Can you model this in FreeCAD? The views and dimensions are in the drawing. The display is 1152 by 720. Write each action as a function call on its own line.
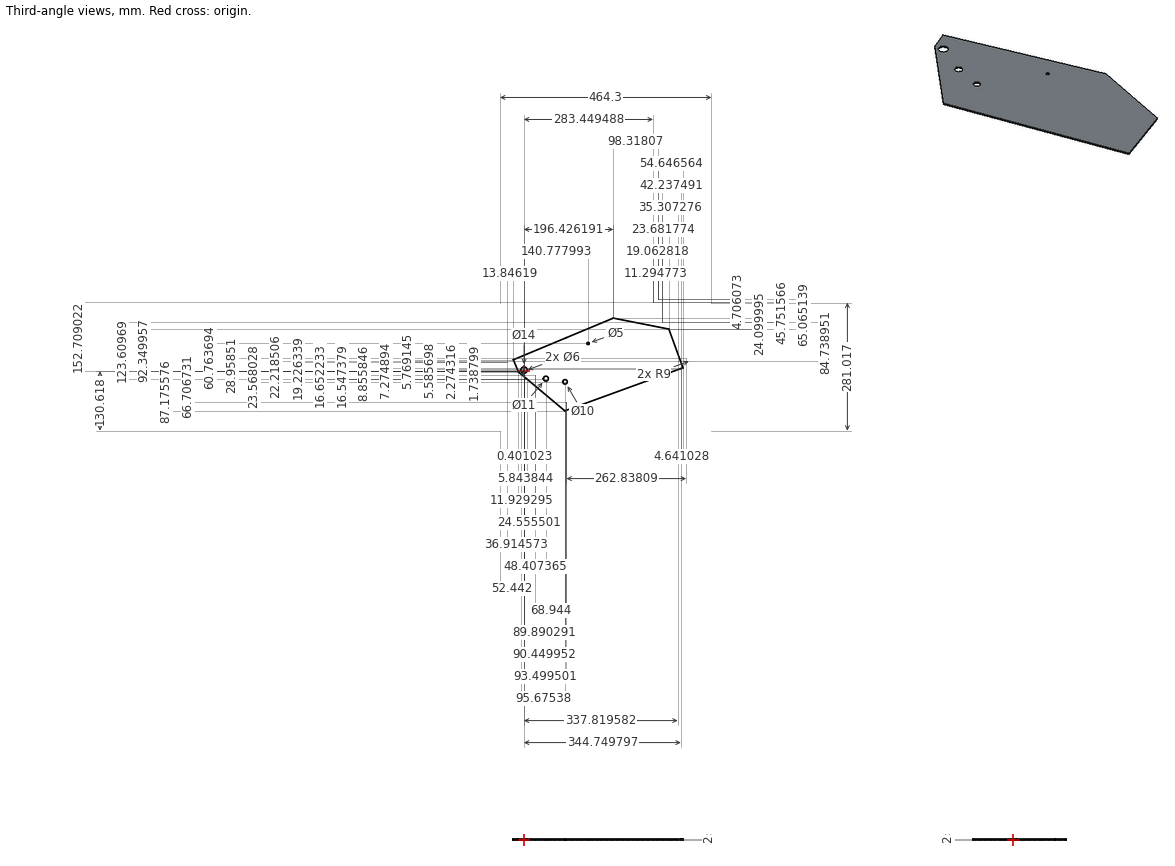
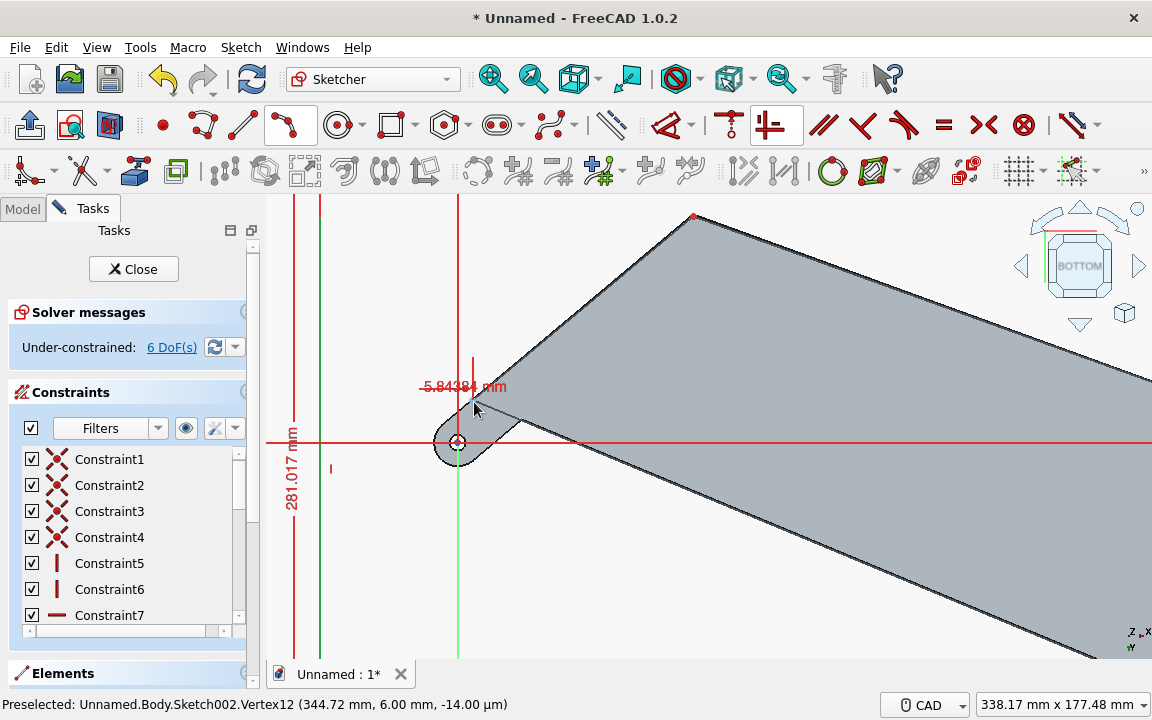
click(473, 400)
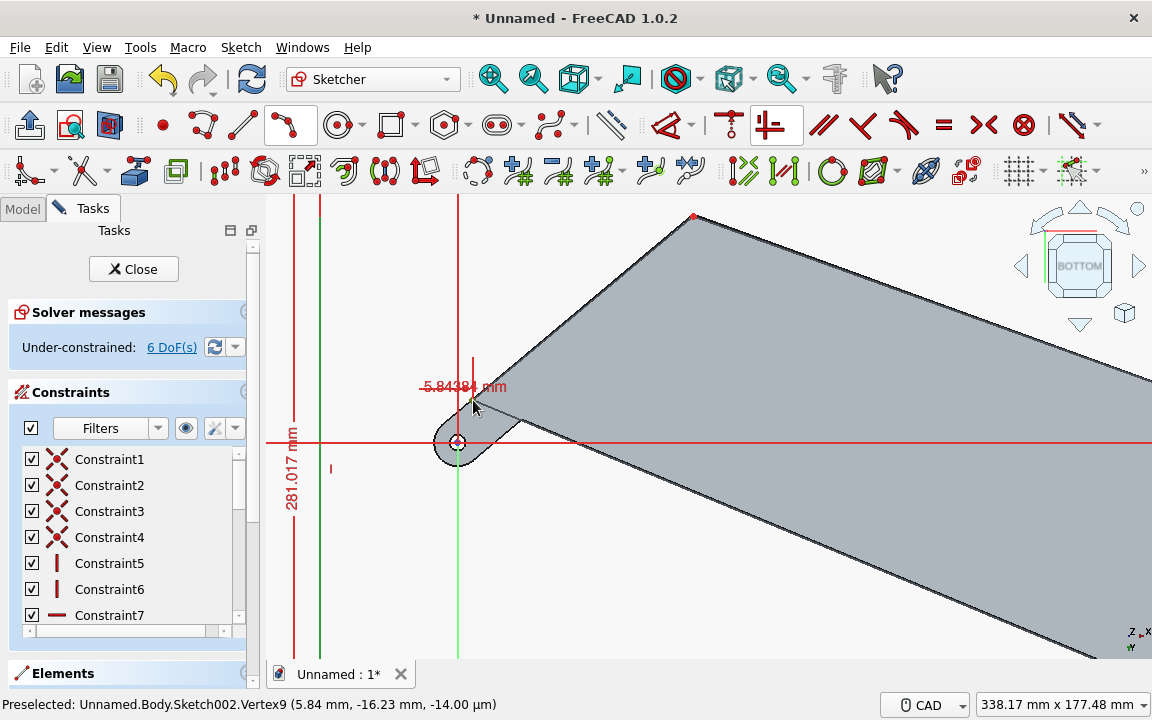
key(i)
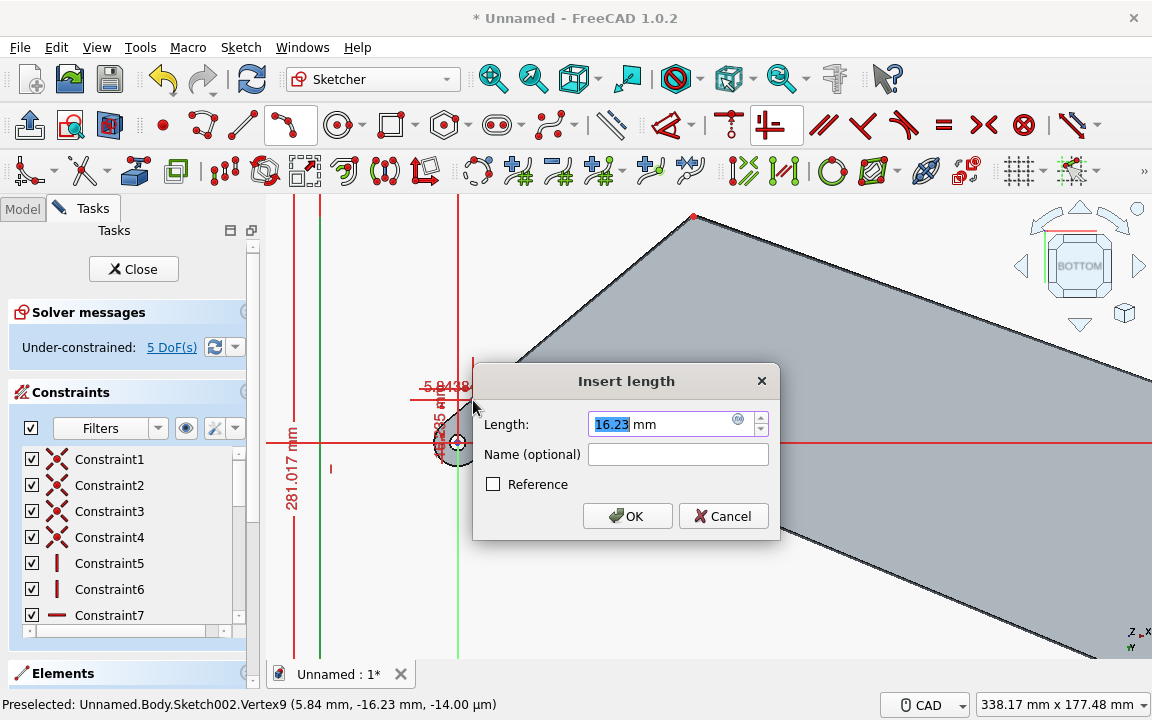
text(16.652233)
key(Return)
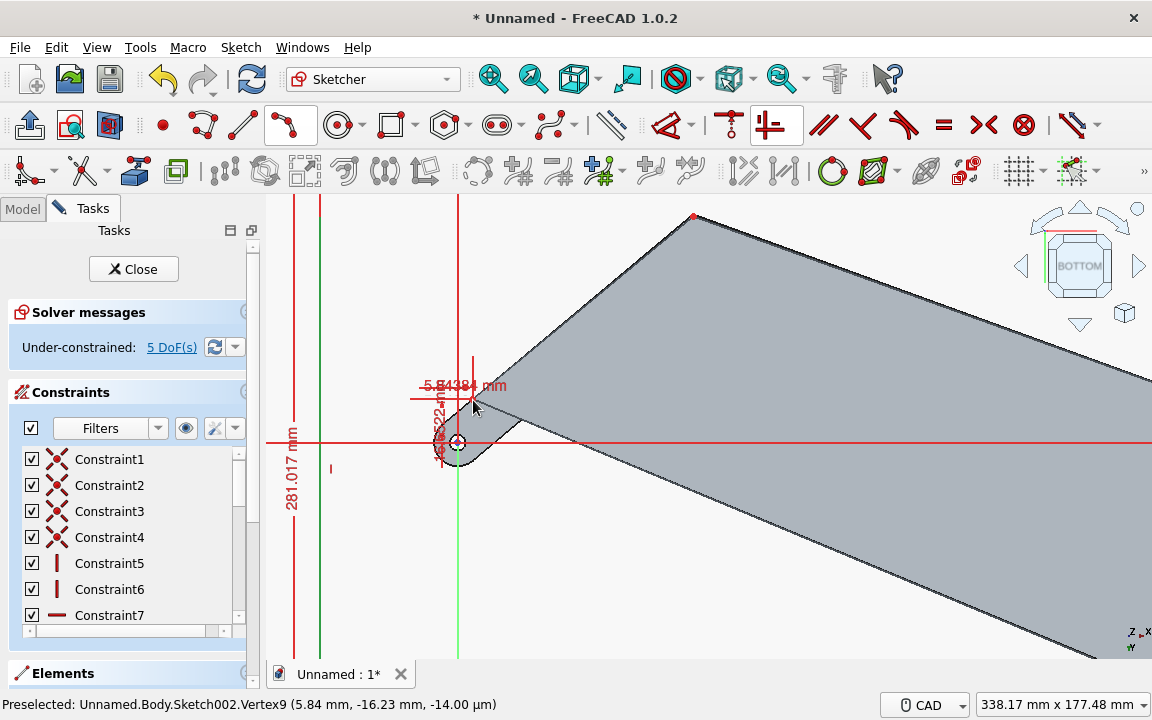
scroll(473, 402, down, 5)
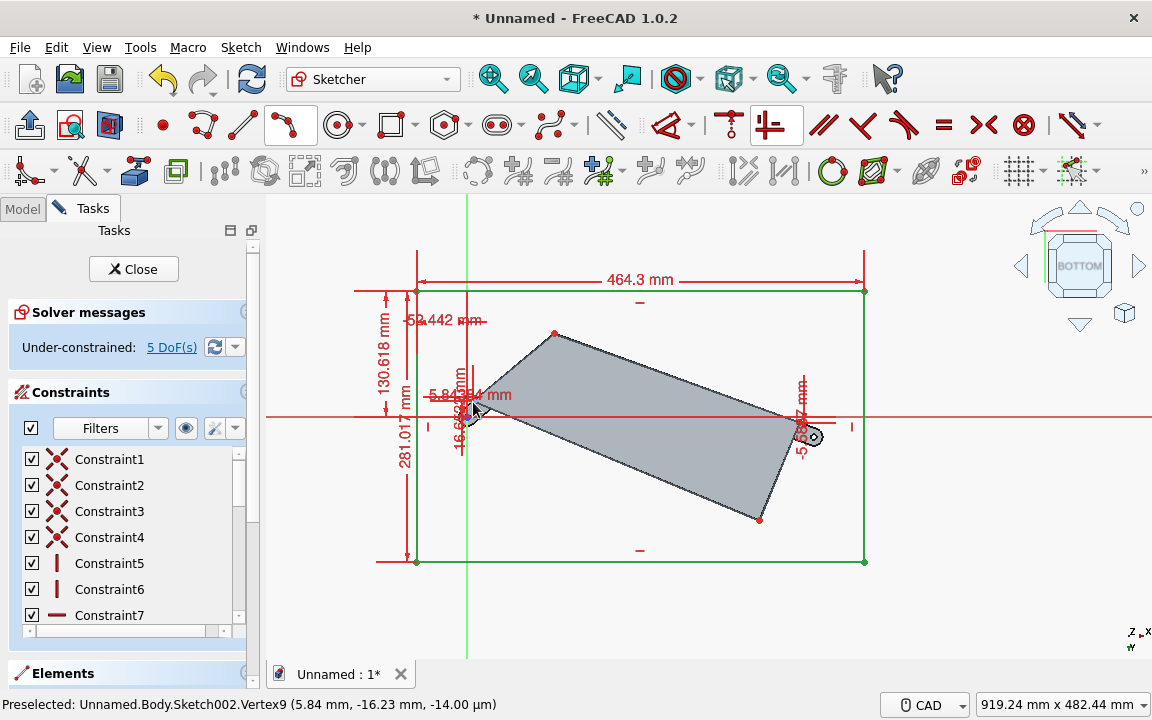
click(554, 334)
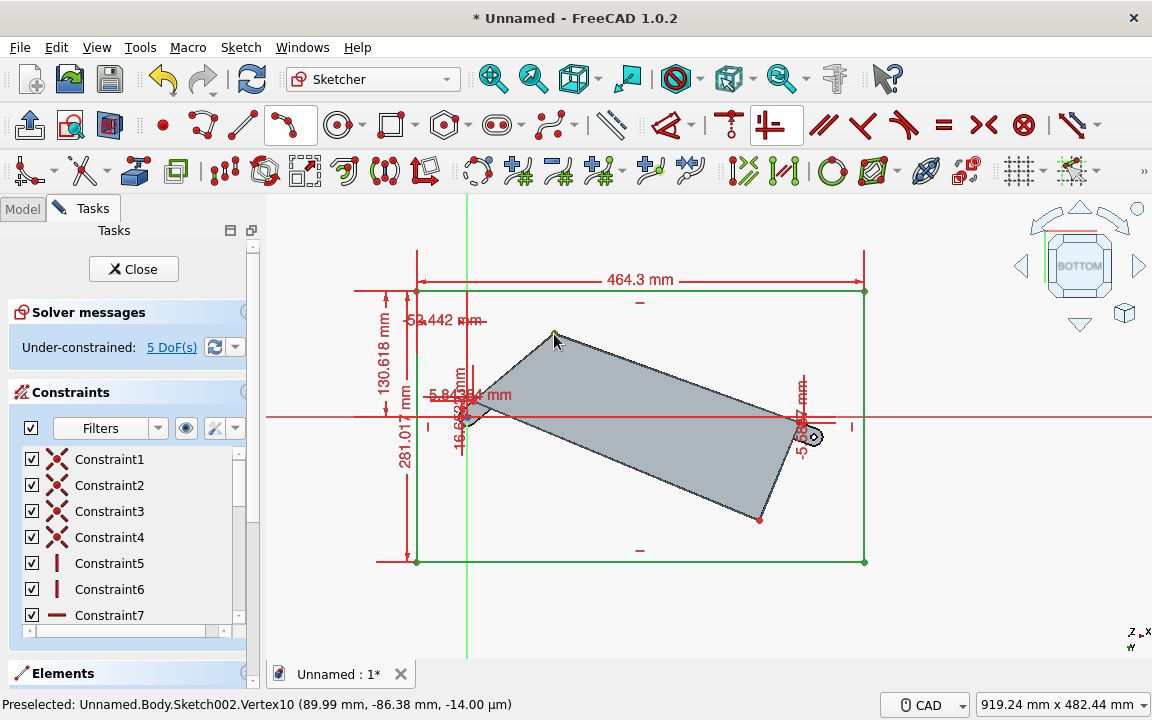
key(l)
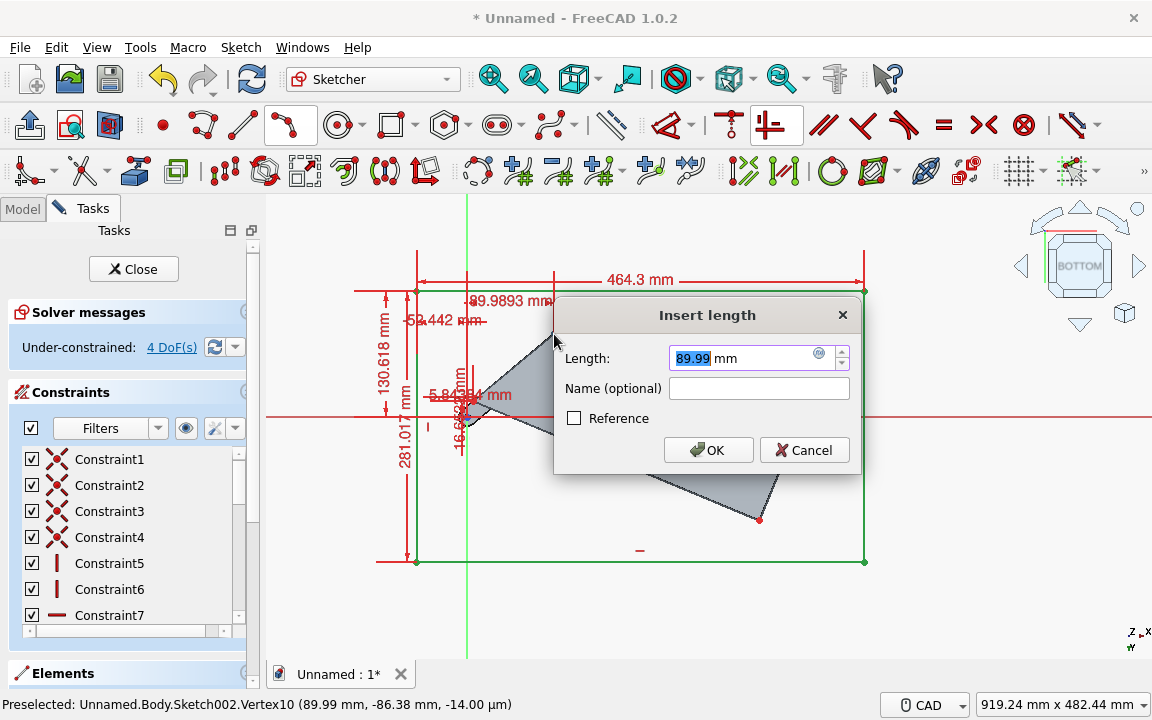
text(89.890291)
key(Return)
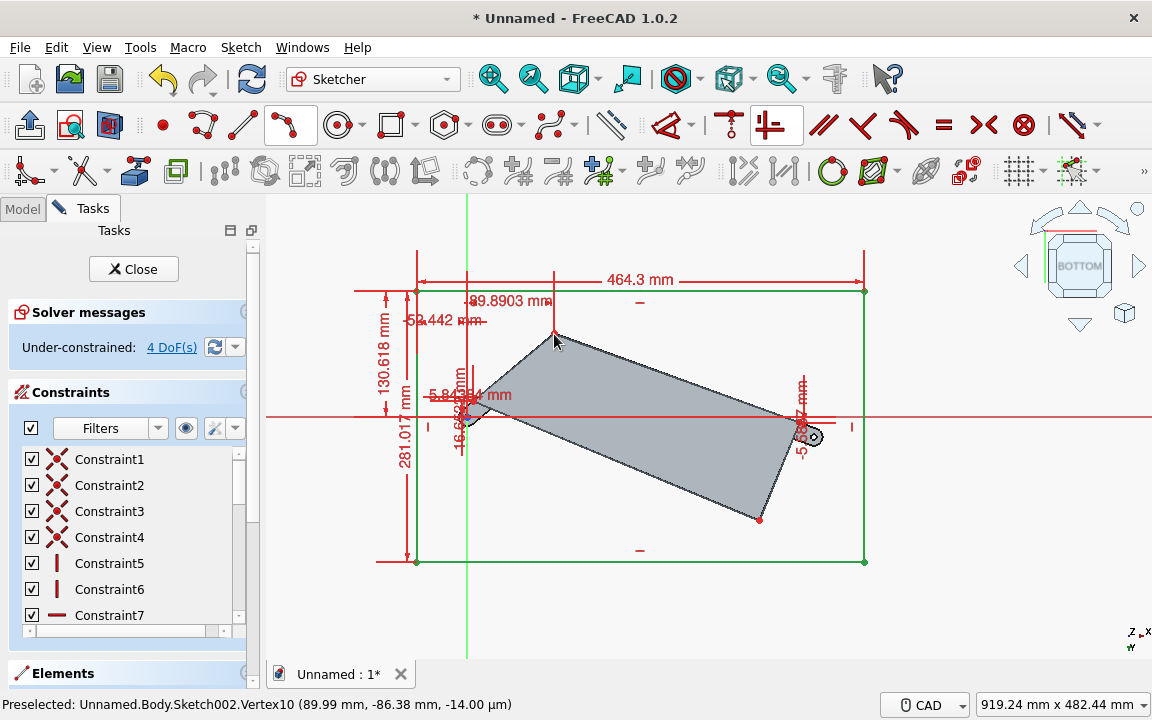
click(554, 334)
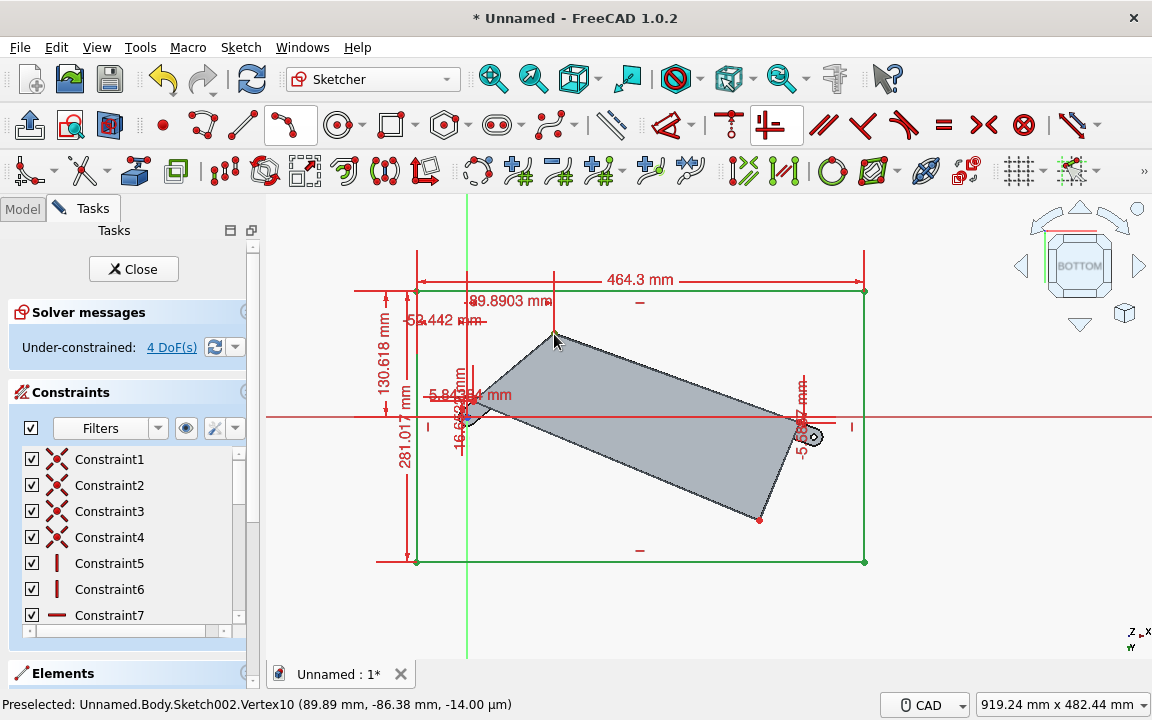
key(i)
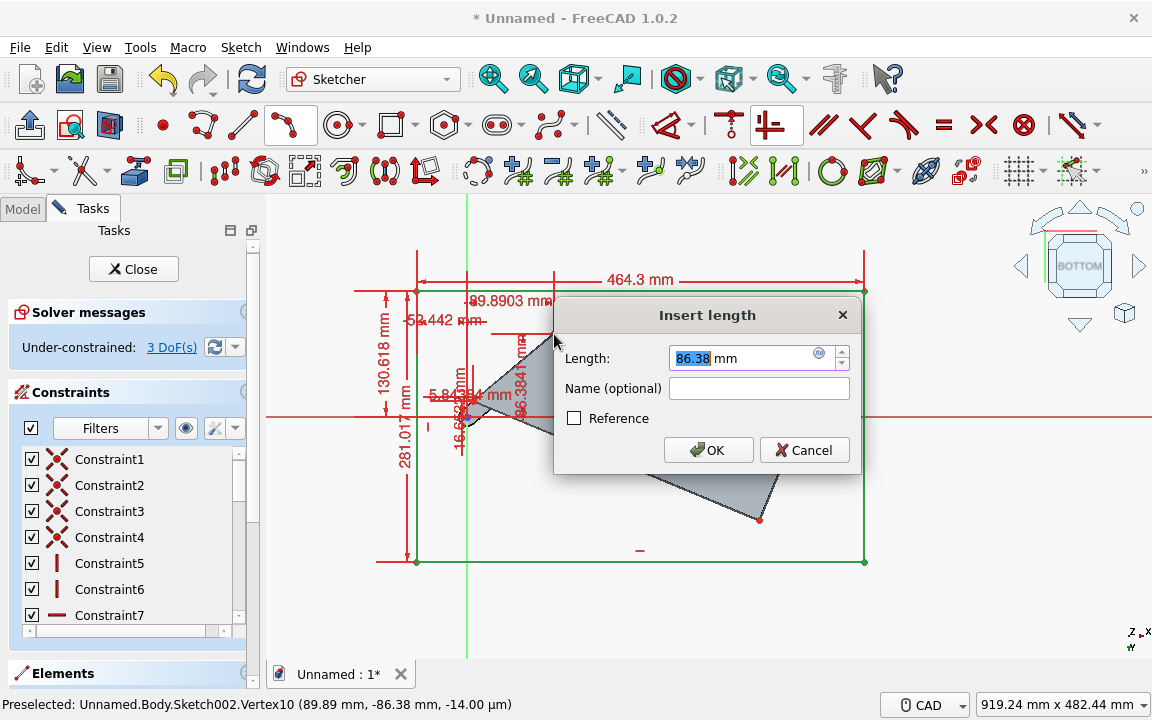
text(87.175576)
key(Return)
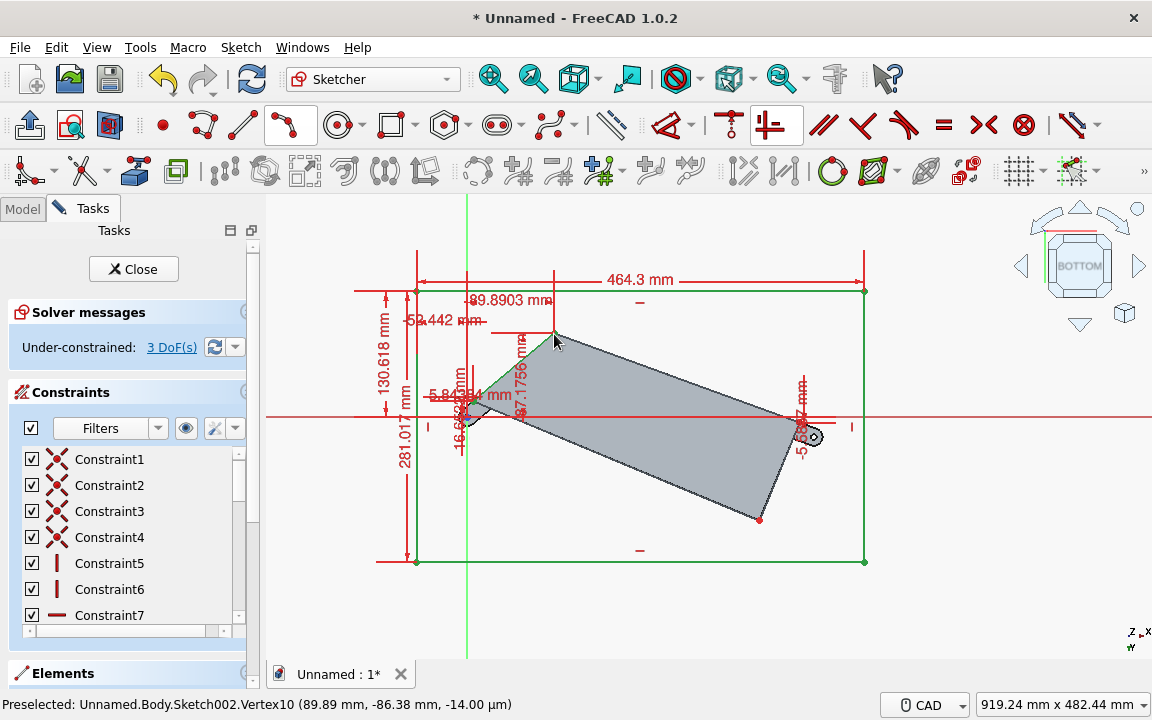
click(788, 452)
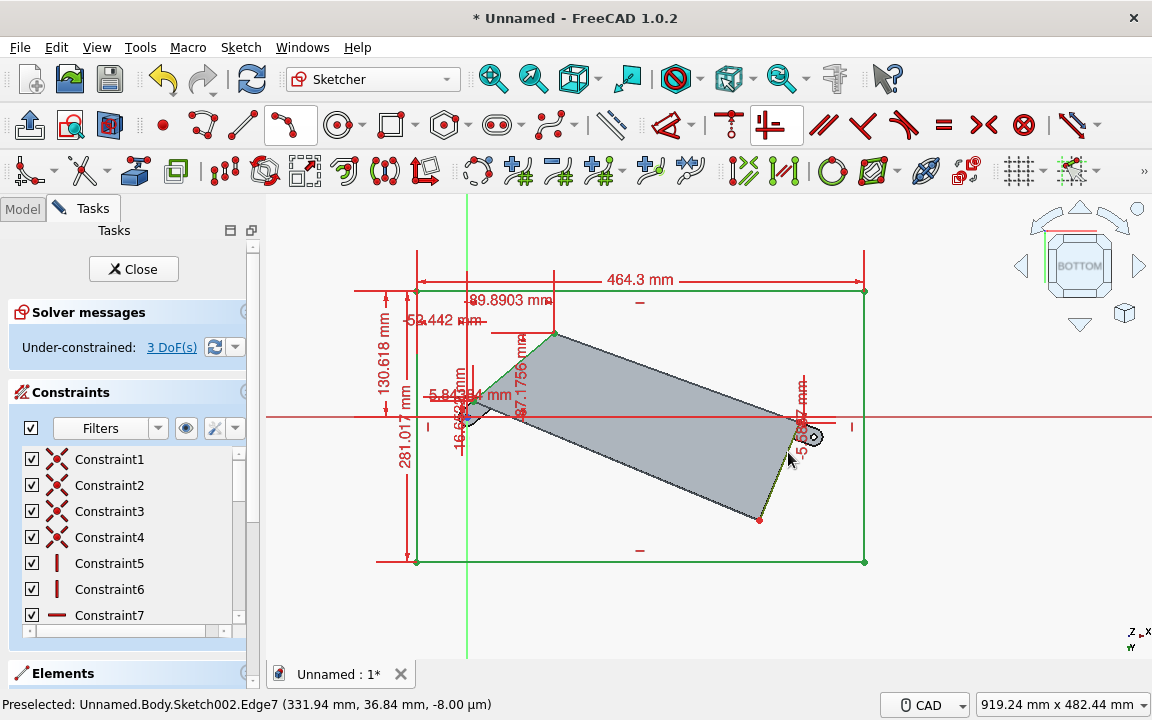
key(l)